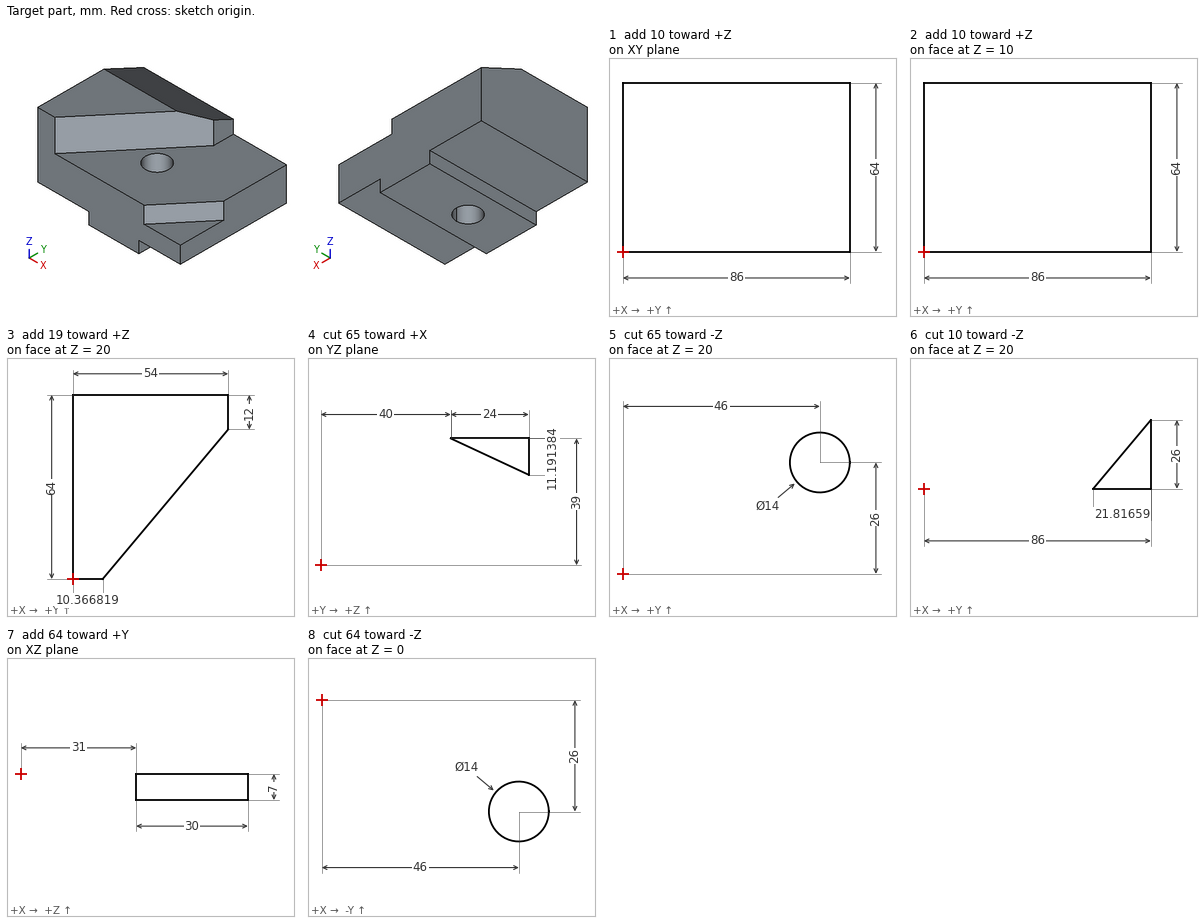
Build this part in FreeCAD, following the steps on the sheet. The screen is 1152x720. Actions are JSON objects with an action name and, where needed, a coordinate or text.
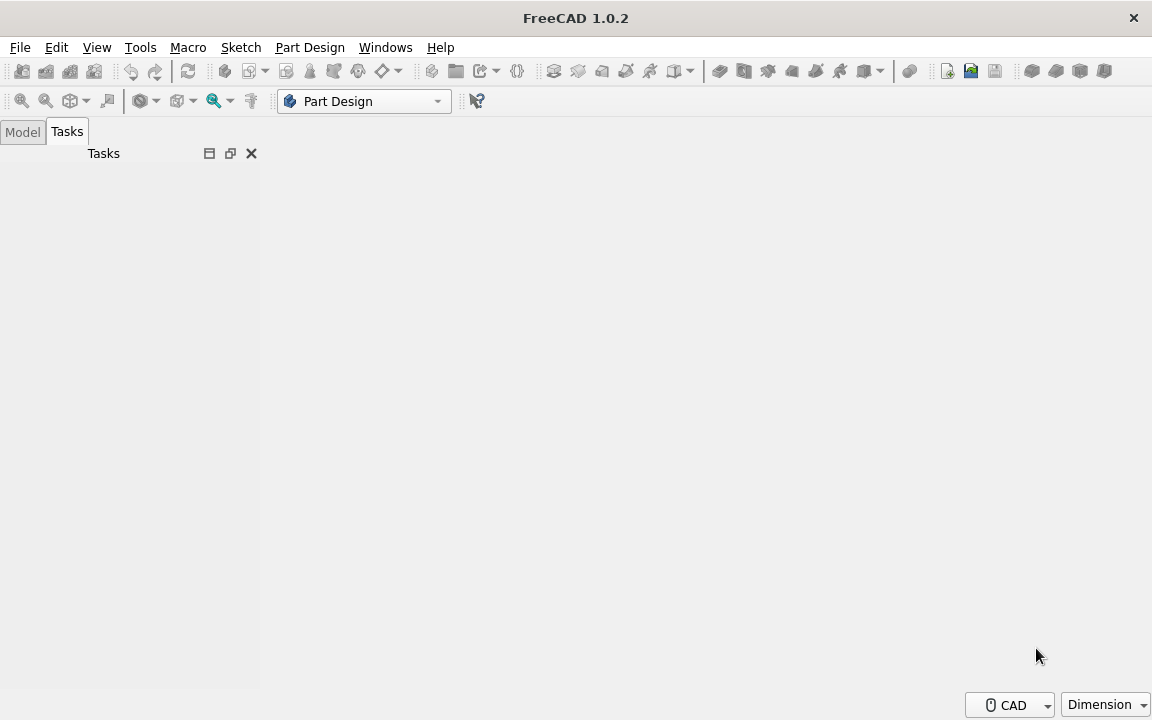
{"action": "left_click", "coordinate": [948, 72]}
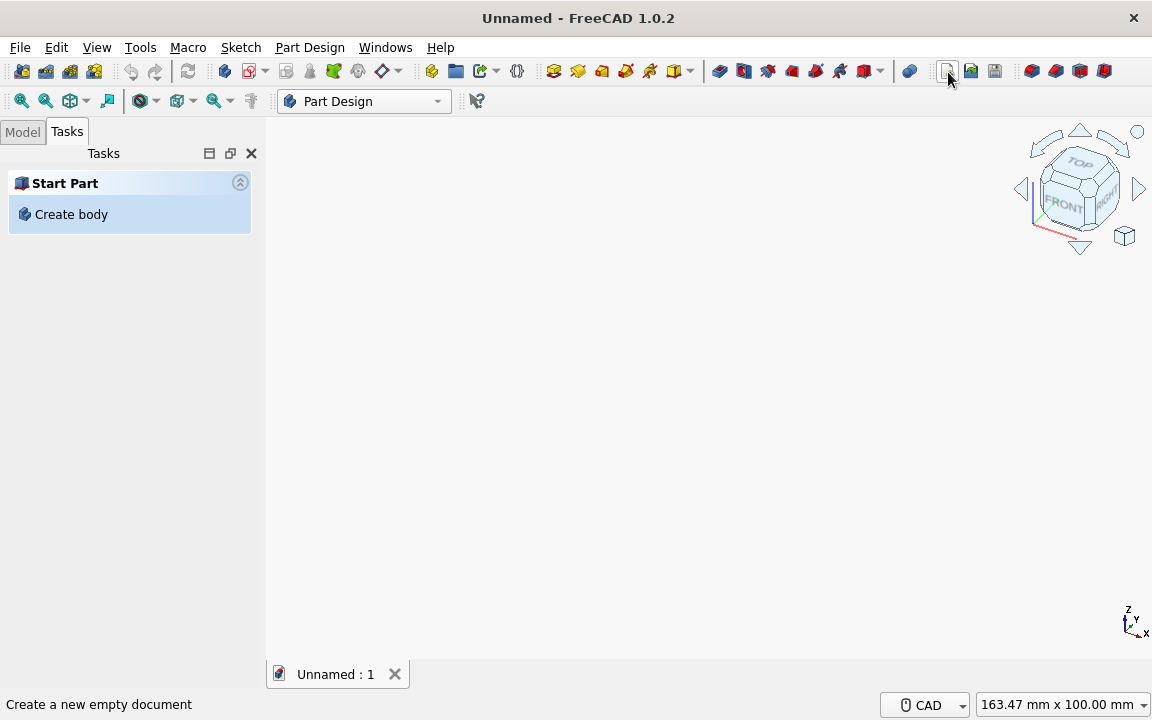
{"action": "left_click", "coordinate": [250, 72]}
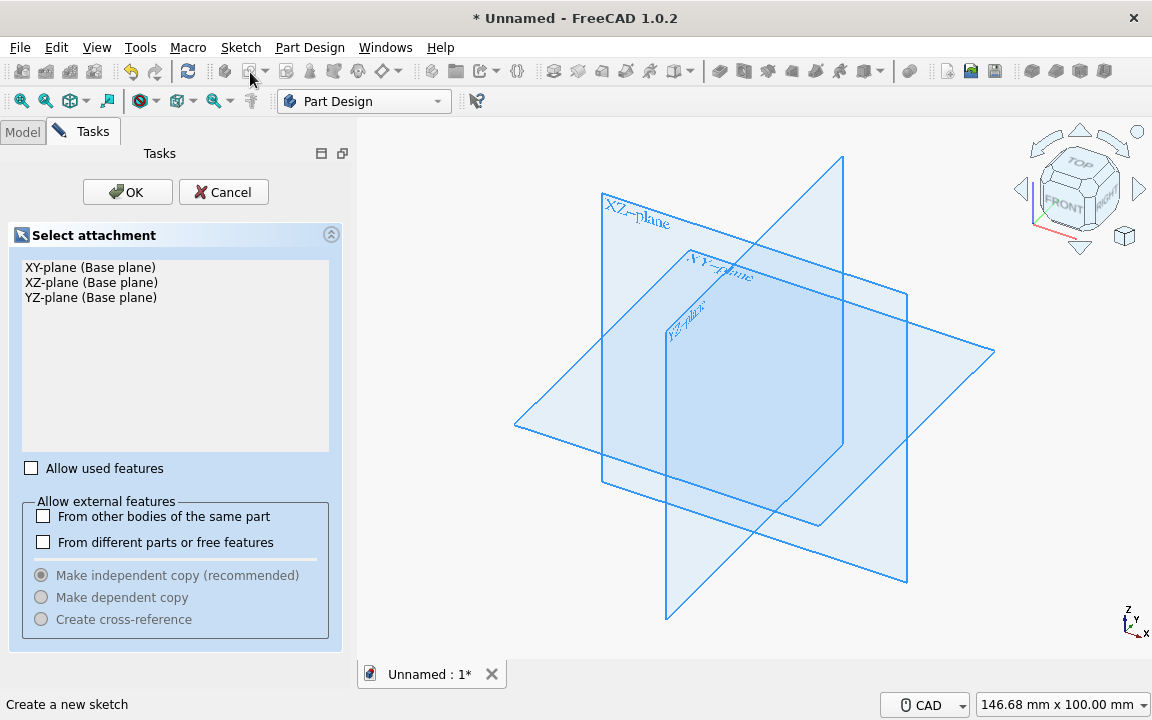
{"action": "left_click", "coordinate": [82, 268]}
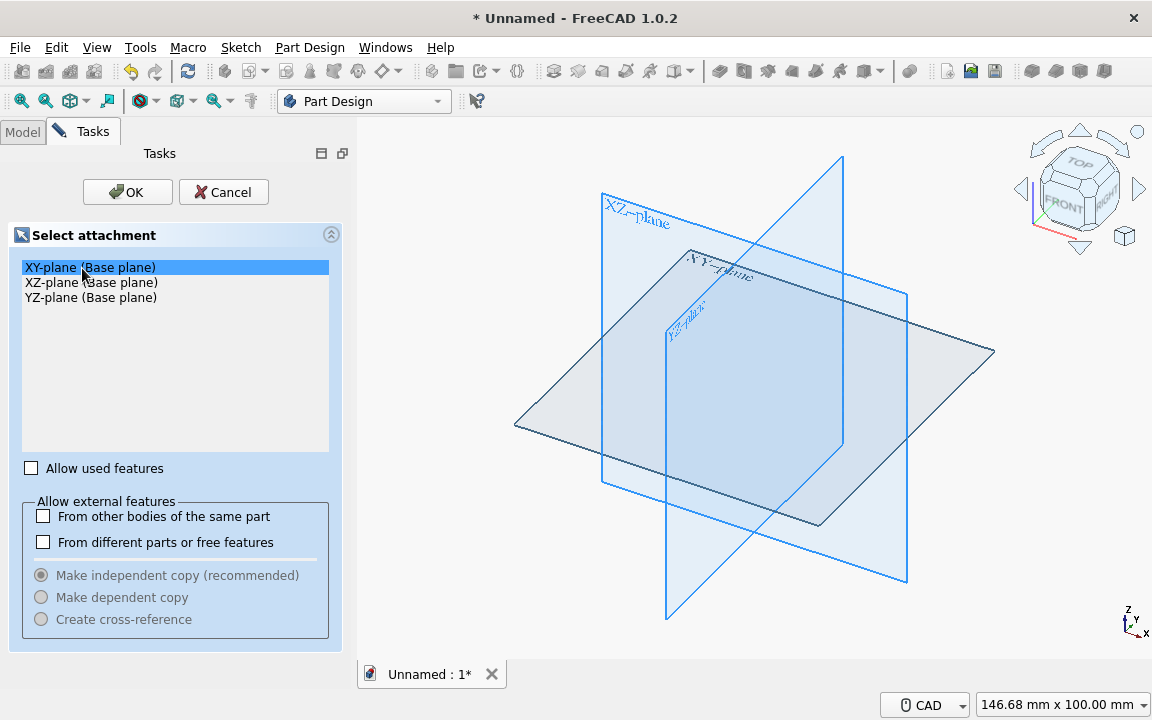
{"action": "left_click", "coordinate": [128, 192]}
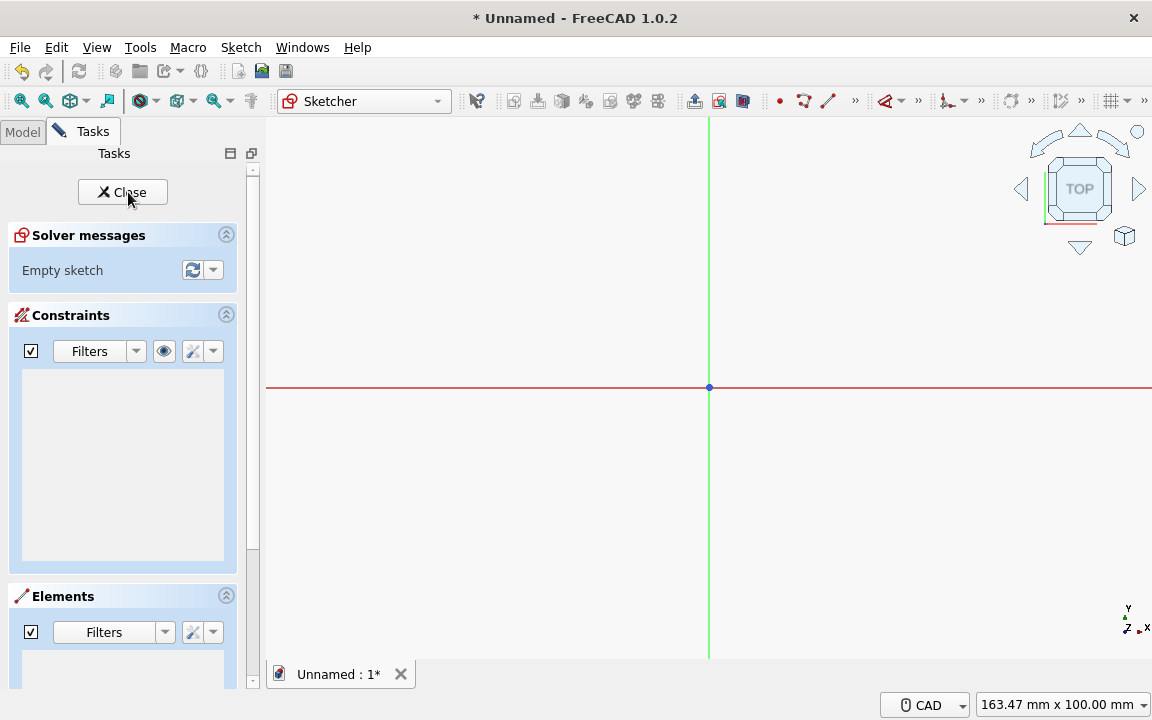
{"action": "scroll", "coordinate": [294, 631], "scroll_direction": "down", "scroll_amount": 2}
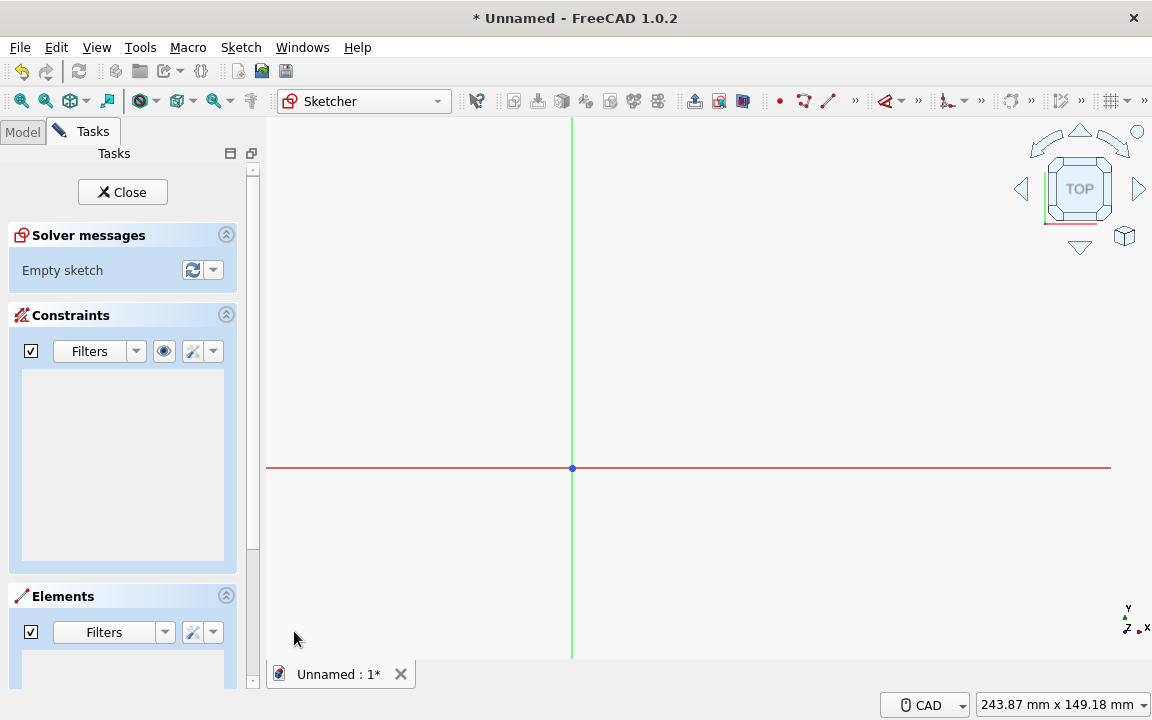
{"action": "scroll", "coordinate": [907, 279], "scroll_direction": "up", "scroll_amount": 2}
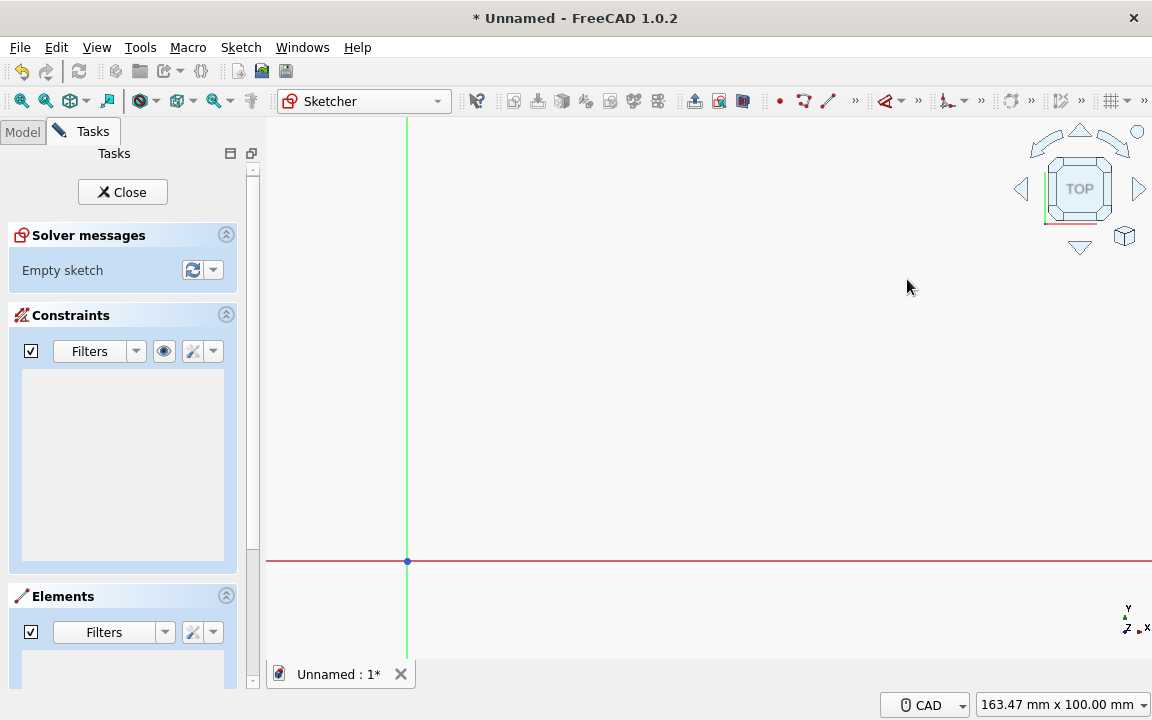
{"action": "key", "text": "g r"}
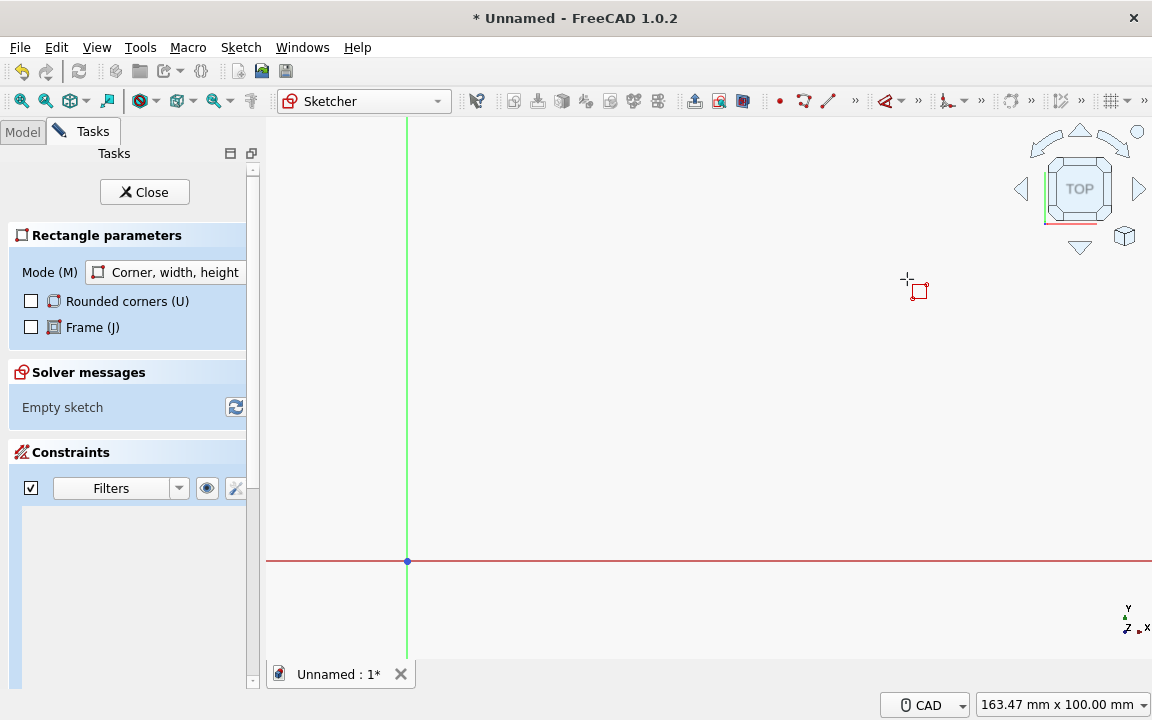
{"action": "left_click", "coordinate": [407, 561]}
{"action": "mouse_move", "coordinate": [873, 215]}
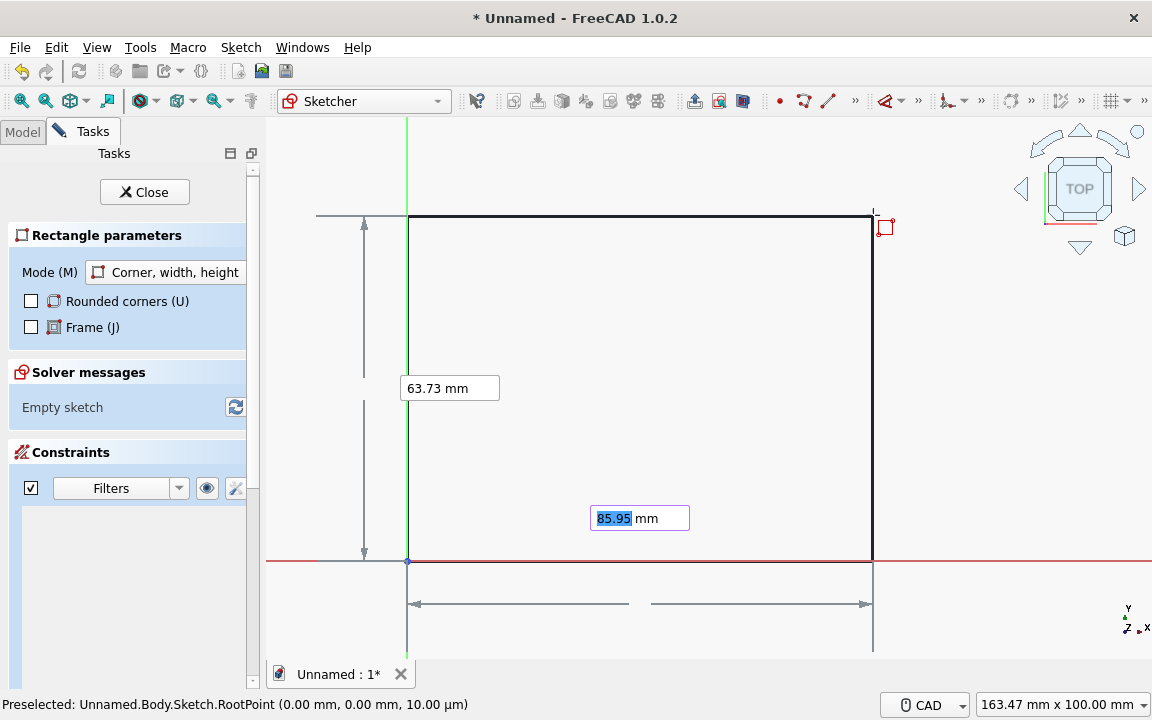
{"action": "type", "text": "86"}
{"action": "key", "text": "Tab"}
{"action": "type", "text": "64"}
{"action": "key", "text": "Return"}
{"action": "key", "text": "Escape"}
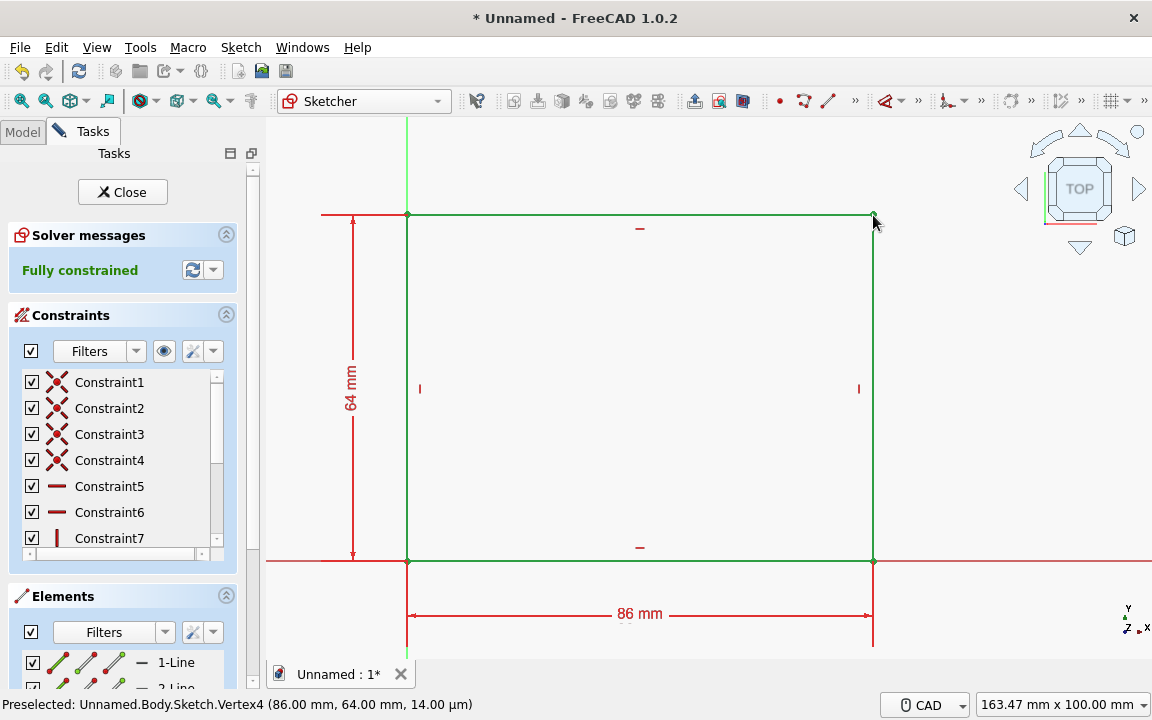
{"action": "left_click", "coordinate": [123, 192]}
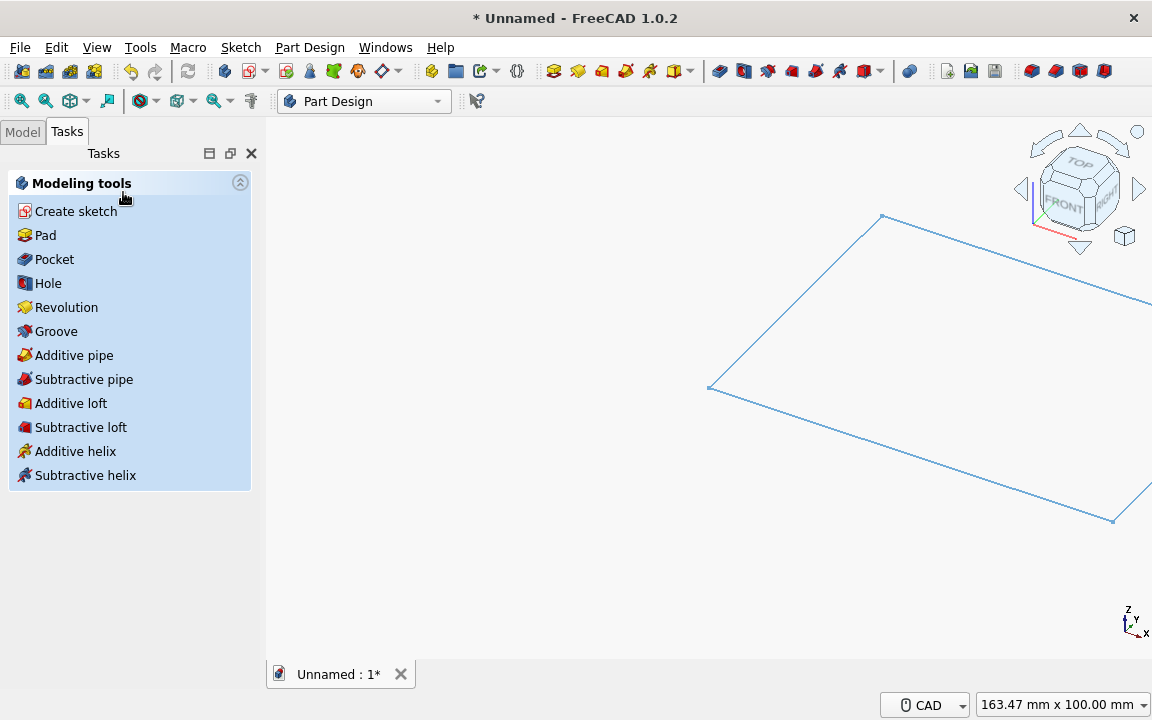
{"action": "left_click", "coordinate": [554, 72]}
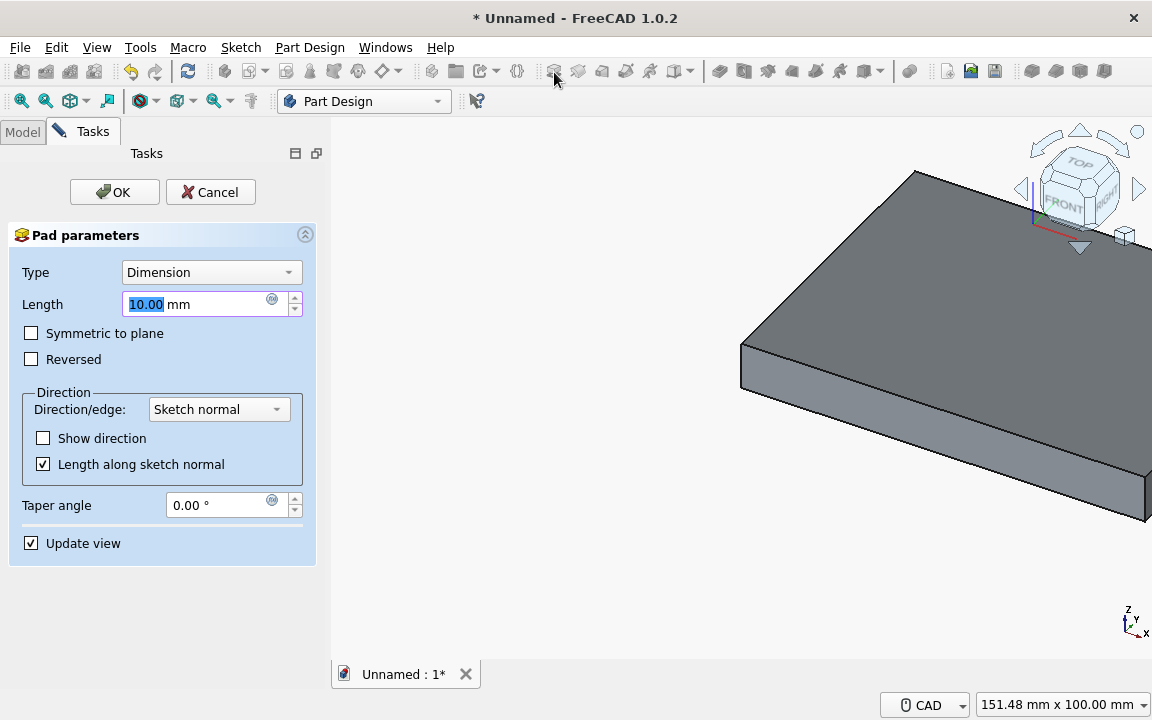
{"action": "type", "text": "10"}
{"action": "key", "text": "Tab"}